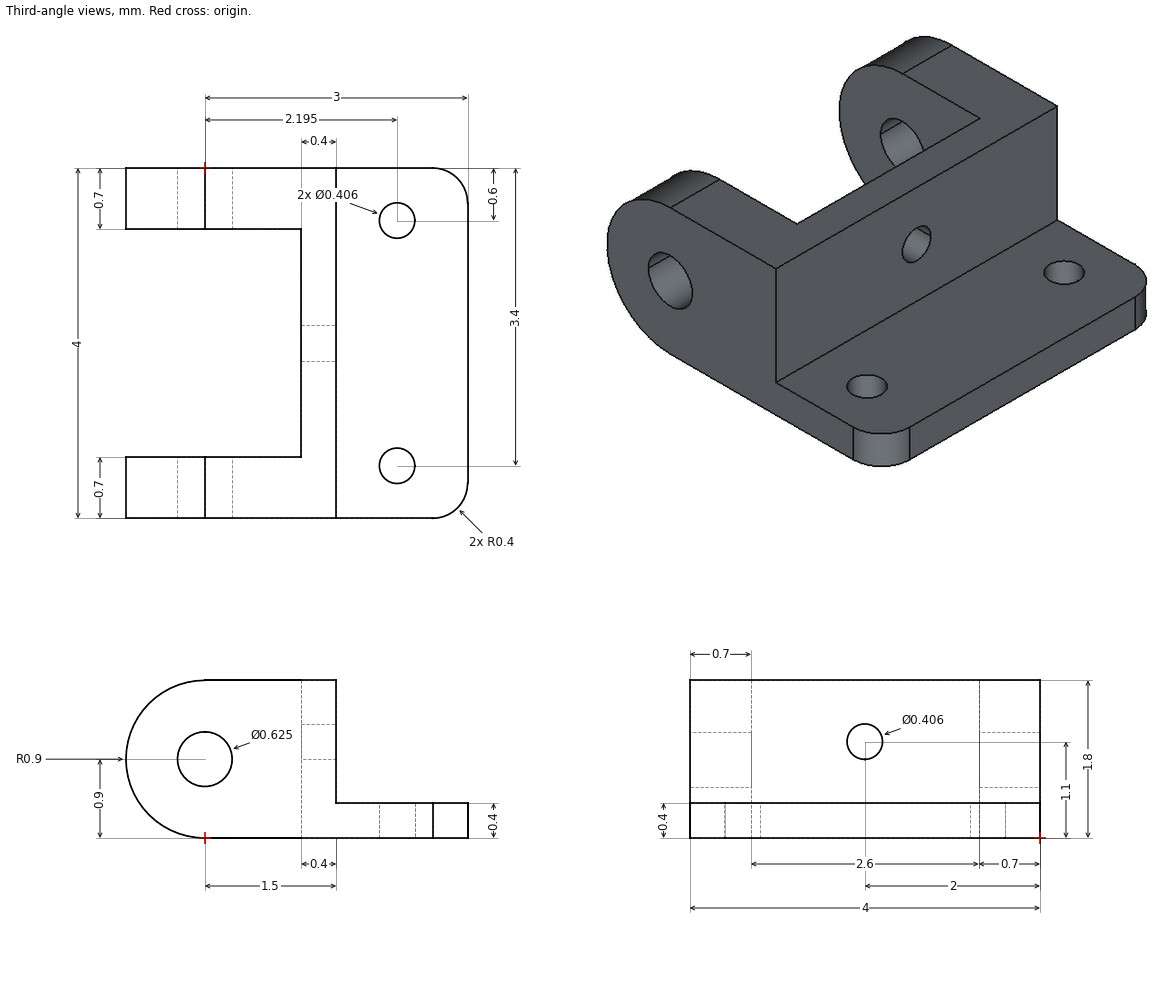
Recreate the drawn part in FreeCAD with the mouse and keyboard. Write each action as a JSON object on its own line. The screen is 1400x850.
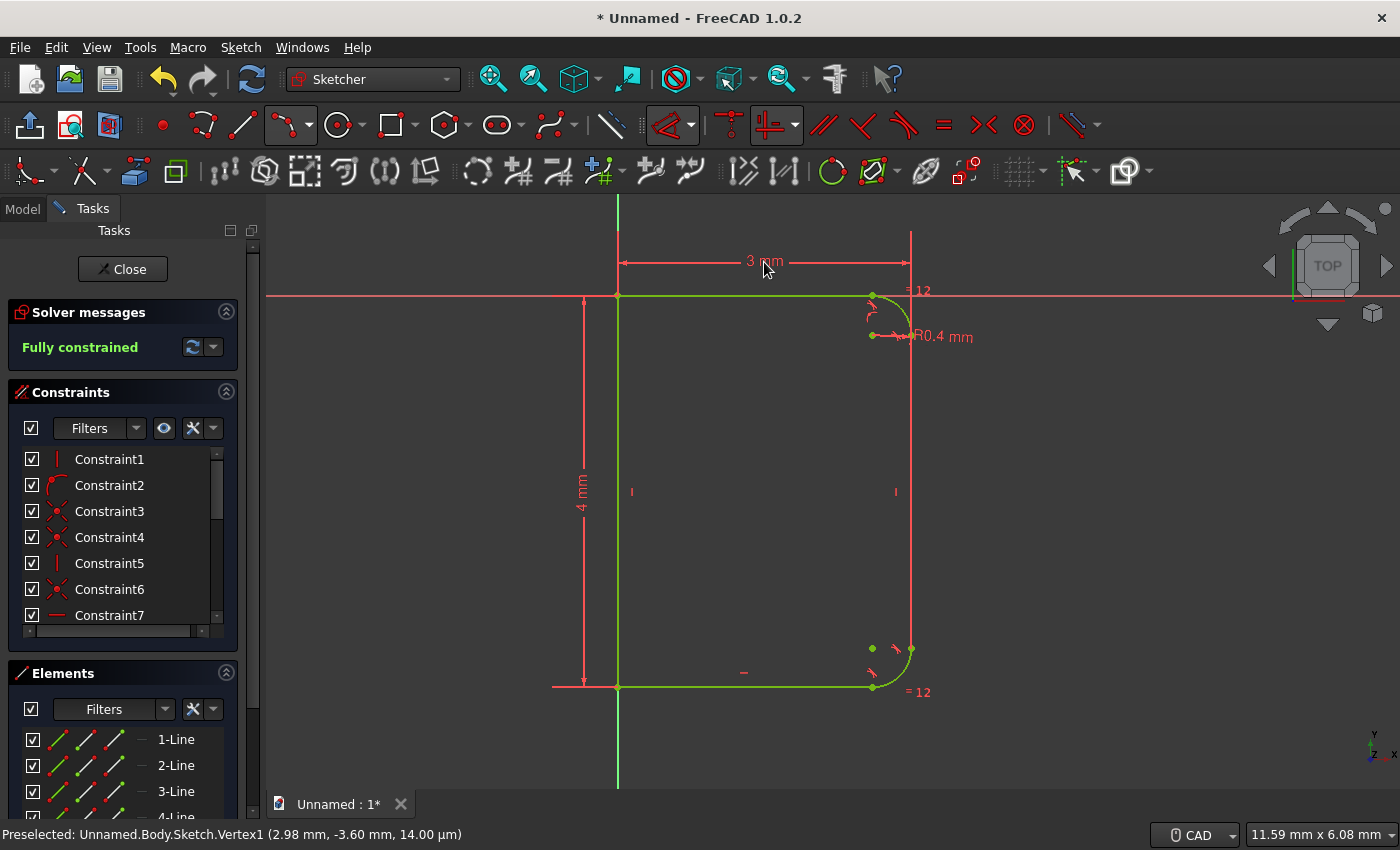
{"action": "left_click", "coordinate": [123, 269]}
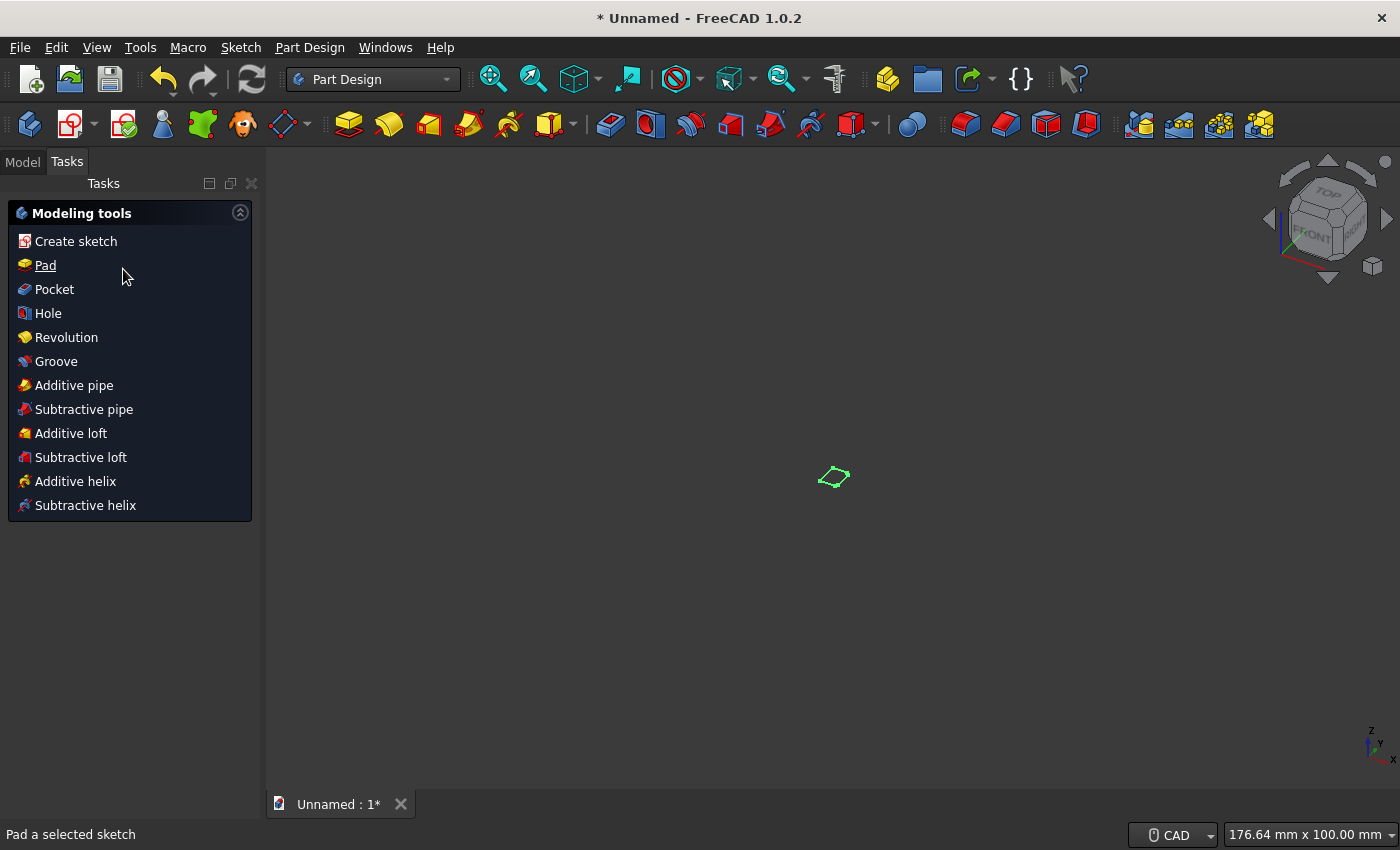
{"action": "left_click", "coordinate": [350, 124]}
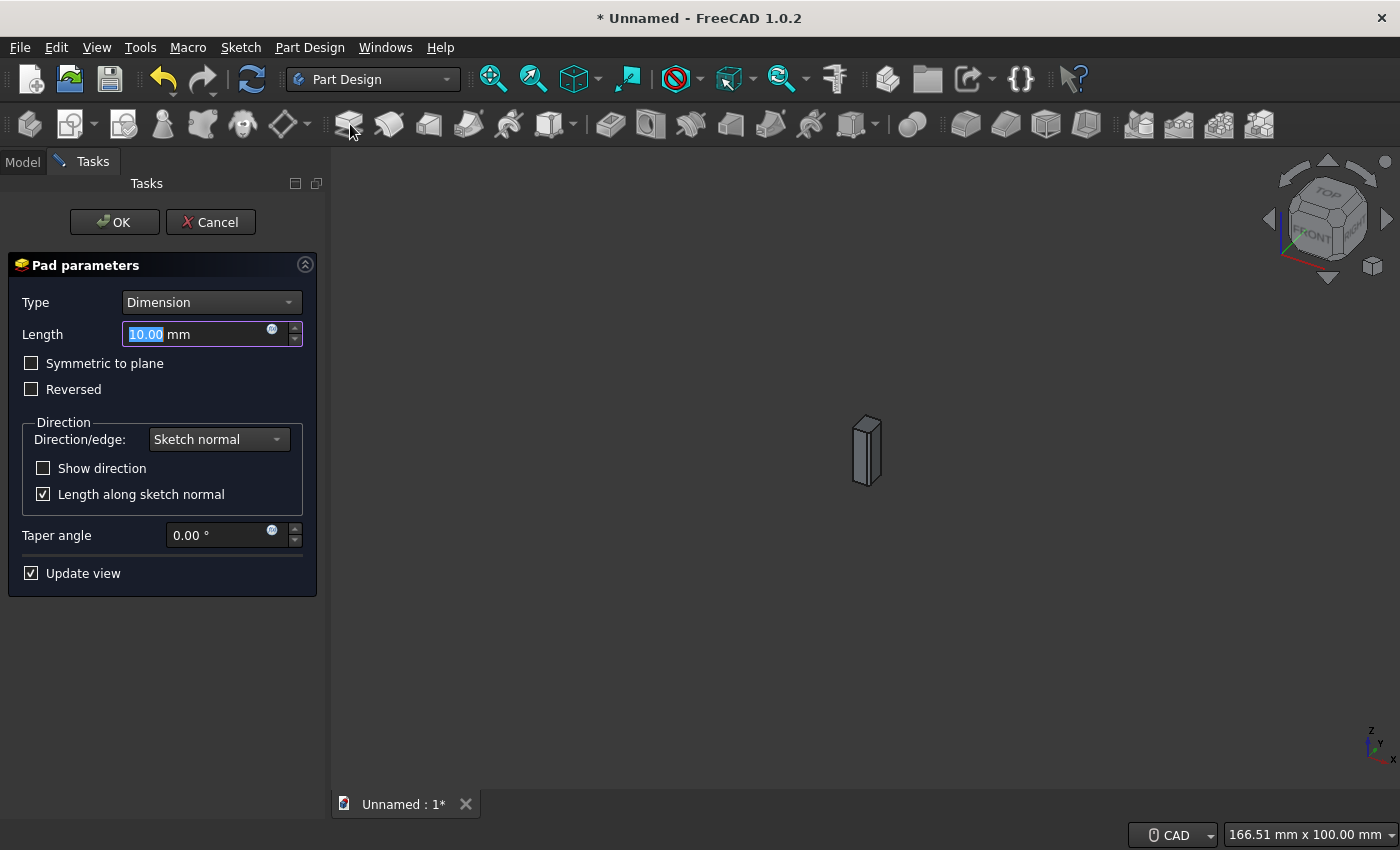
{"action": "type", "text": "0.4"}
{"action": "key", "text": "Tab"}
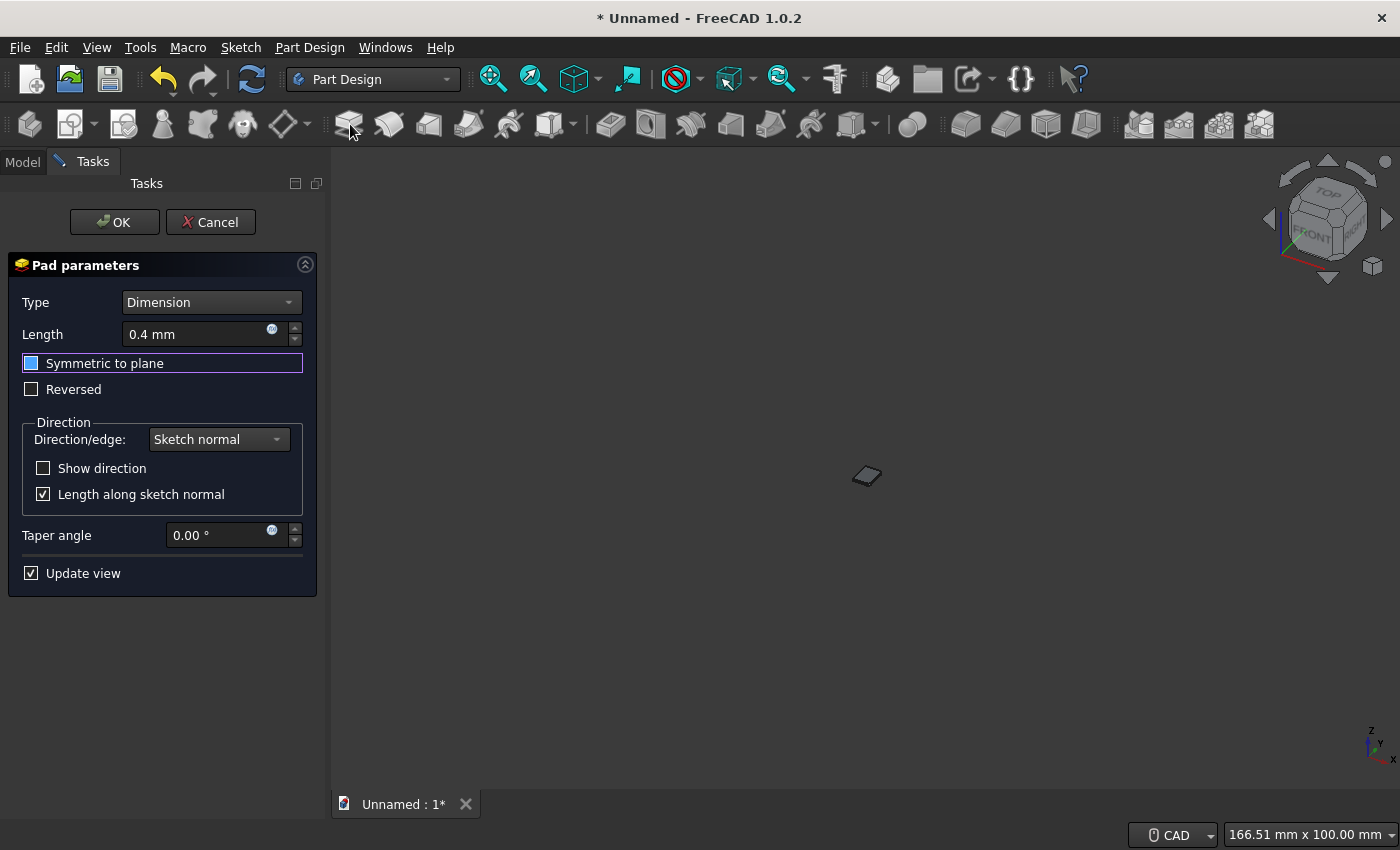
{"action": "left_click", "coordinate": [115, 222]}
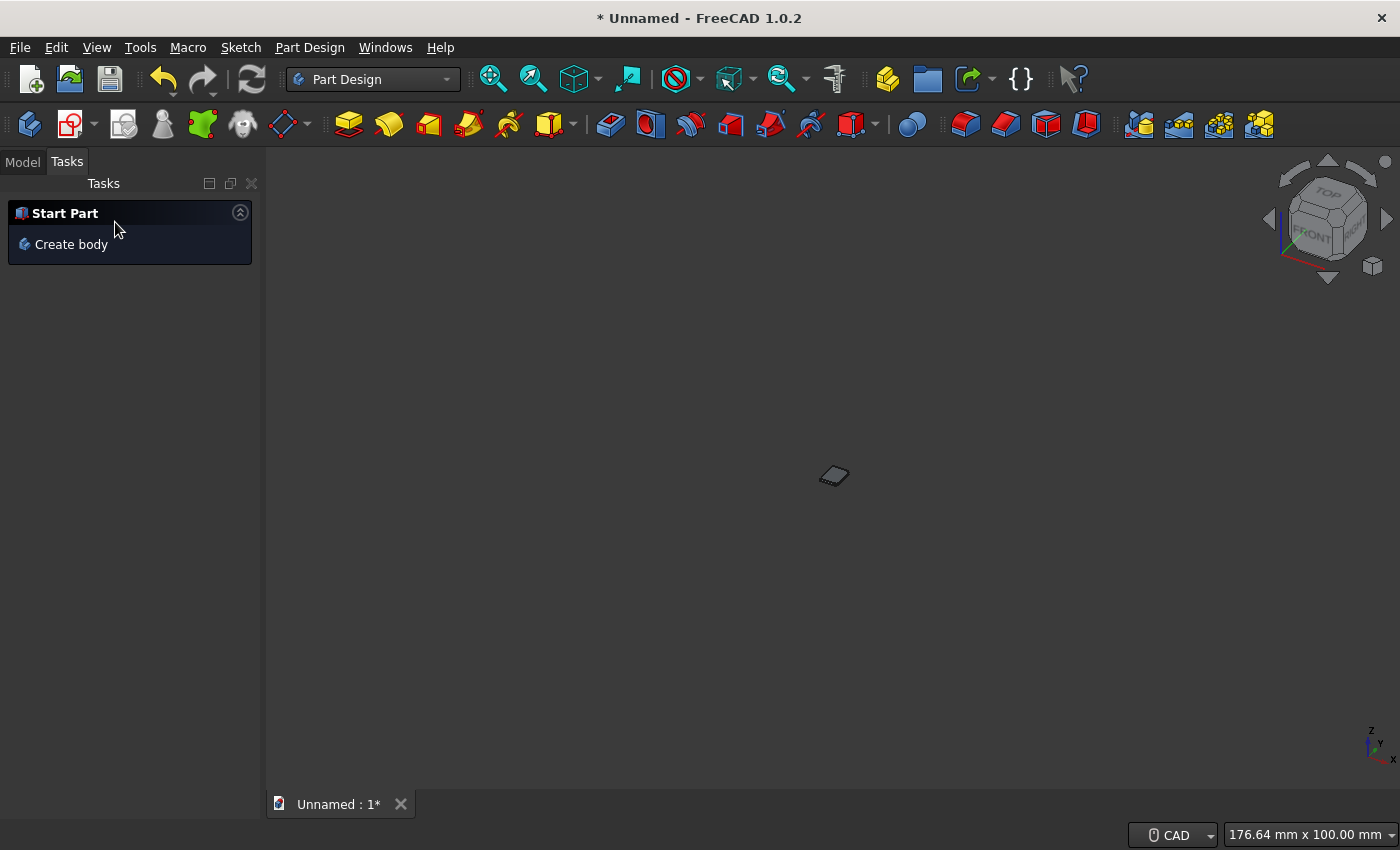
{"action": "key", "text": "v f"}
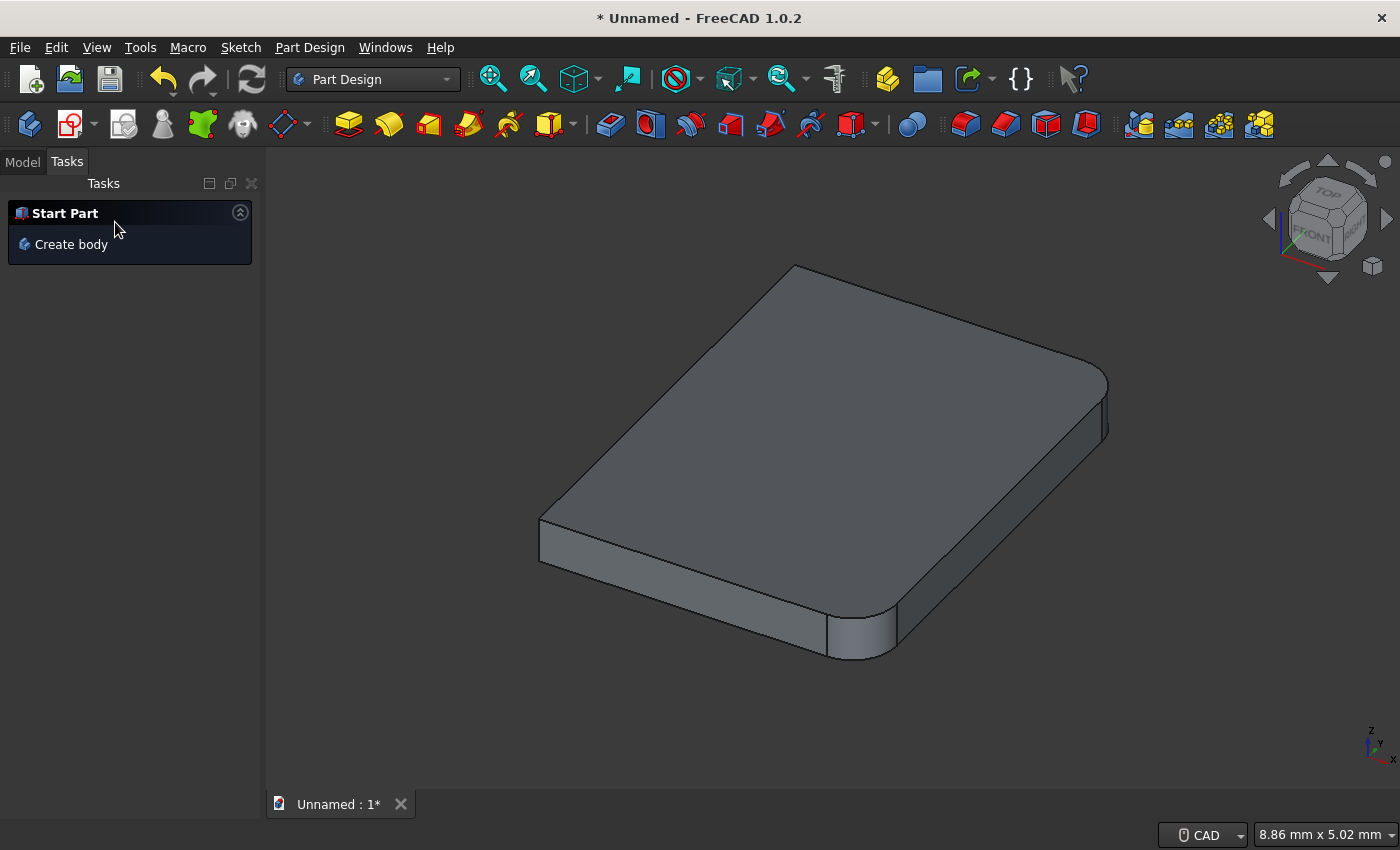
{"action": "left_click", "coordinate": [70, 124]}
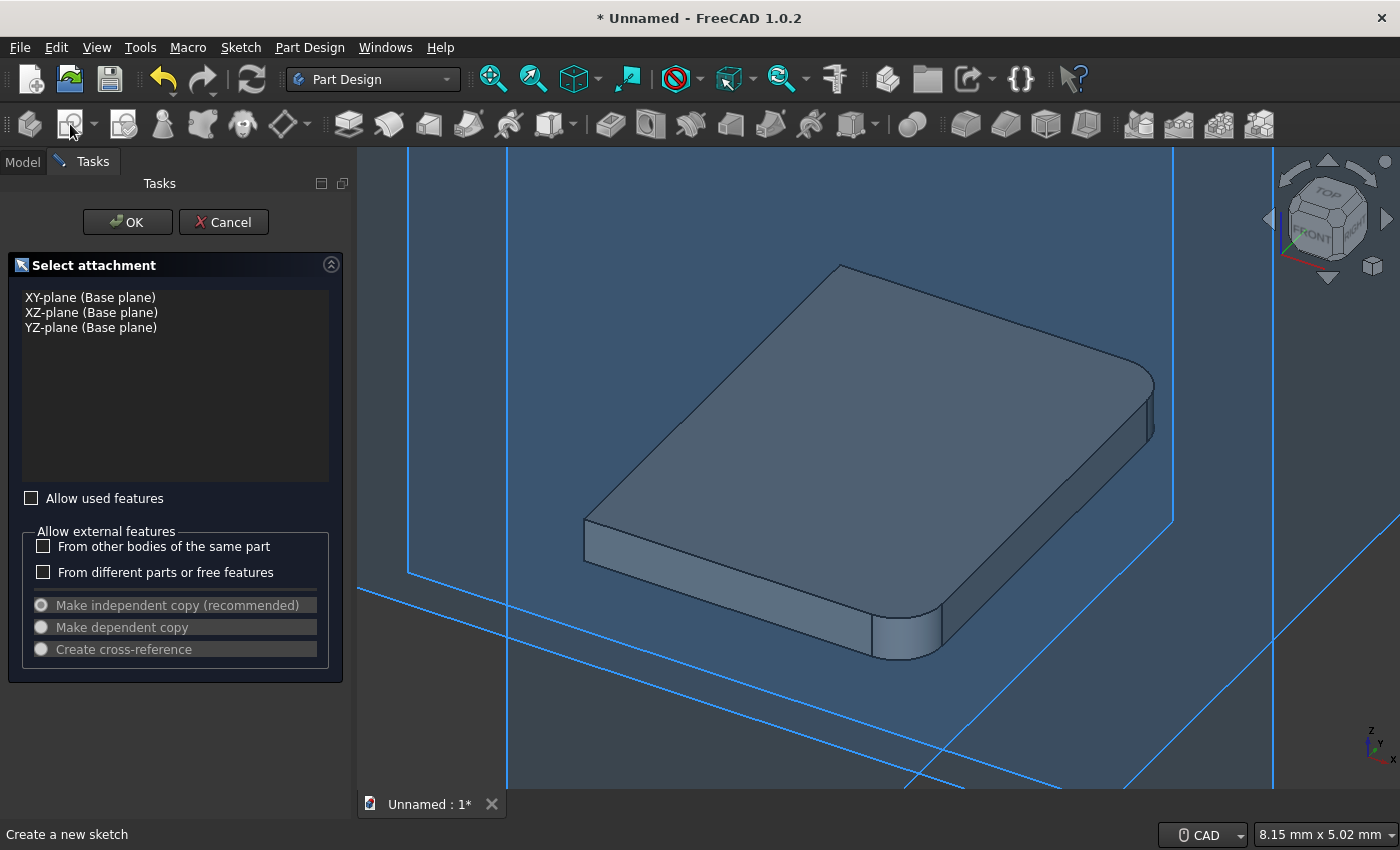
{"action": "left_click", "coordinate": [82, 328]}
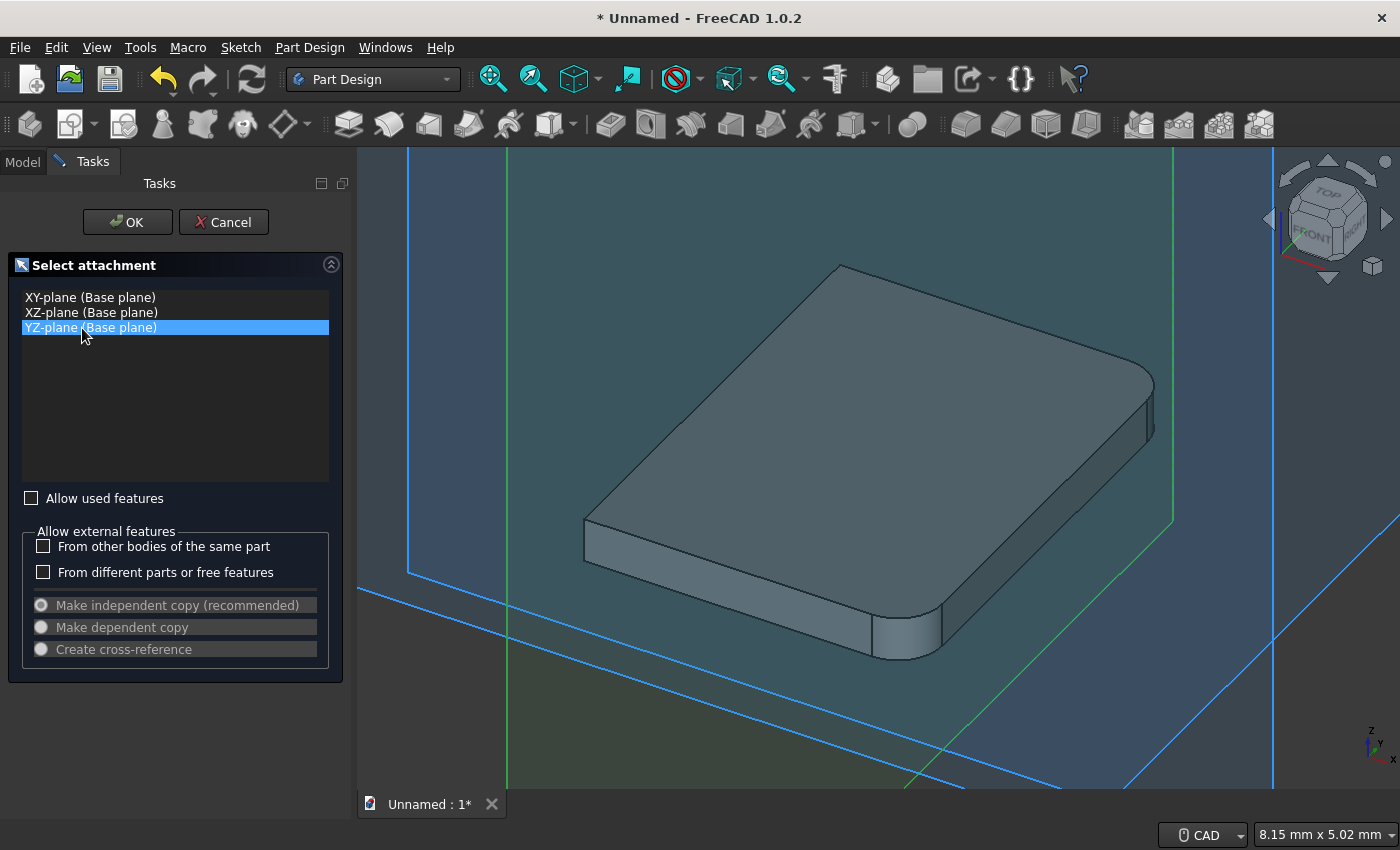
{"action": "left_click", "coordinate": [128, 222]}